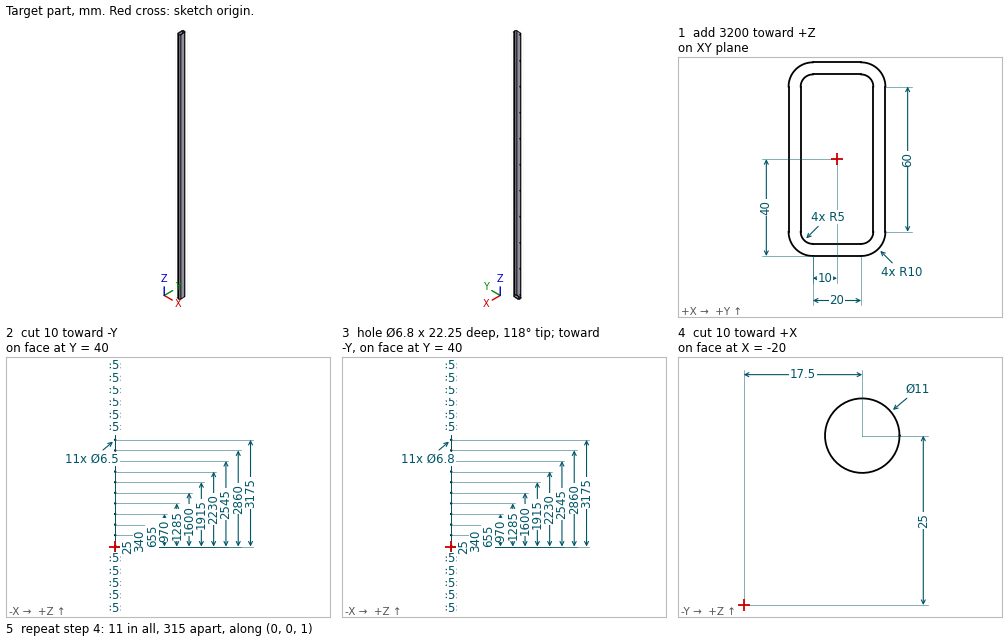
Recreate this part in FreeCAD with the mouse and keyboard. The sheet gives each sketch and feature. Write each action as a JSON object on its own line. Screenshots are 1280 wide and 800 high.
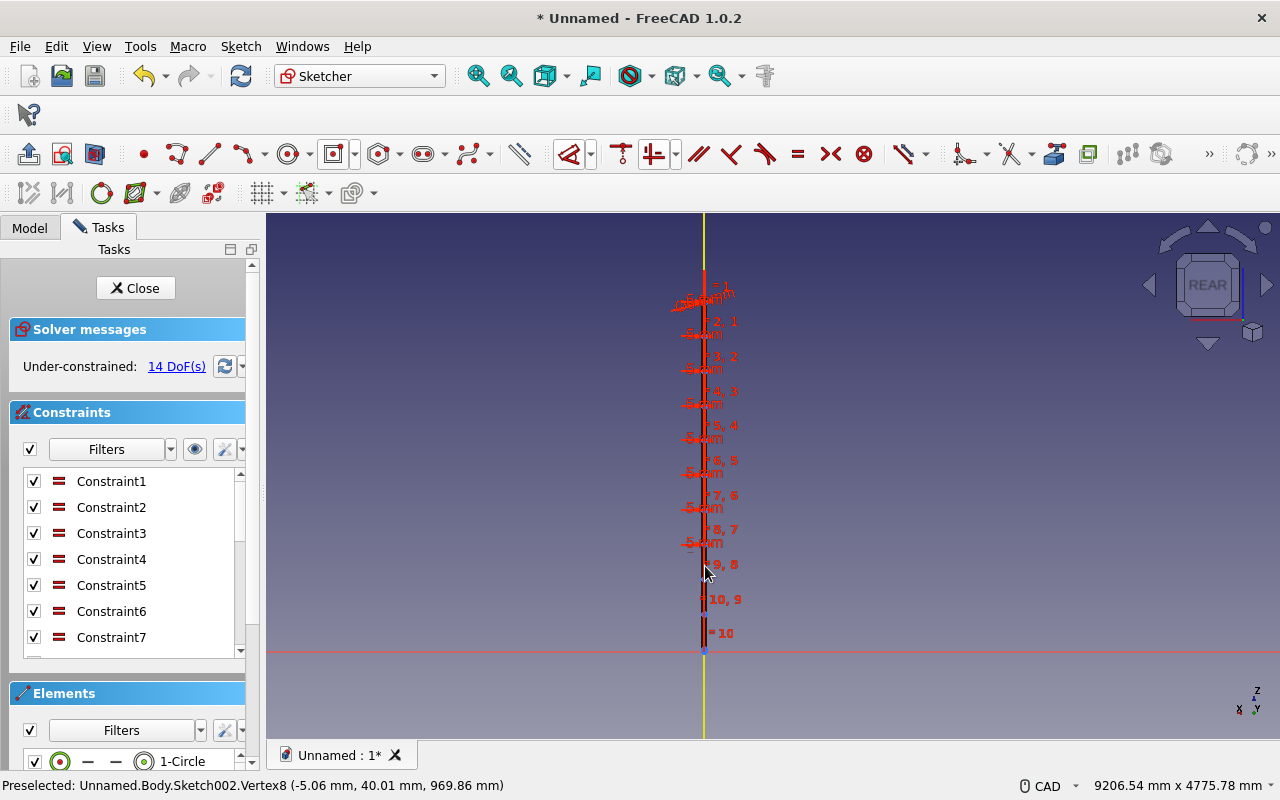
{"action": "scroll", "coordinate": [705, 580], "scroll_direction": "up", "scroll_amount": 22}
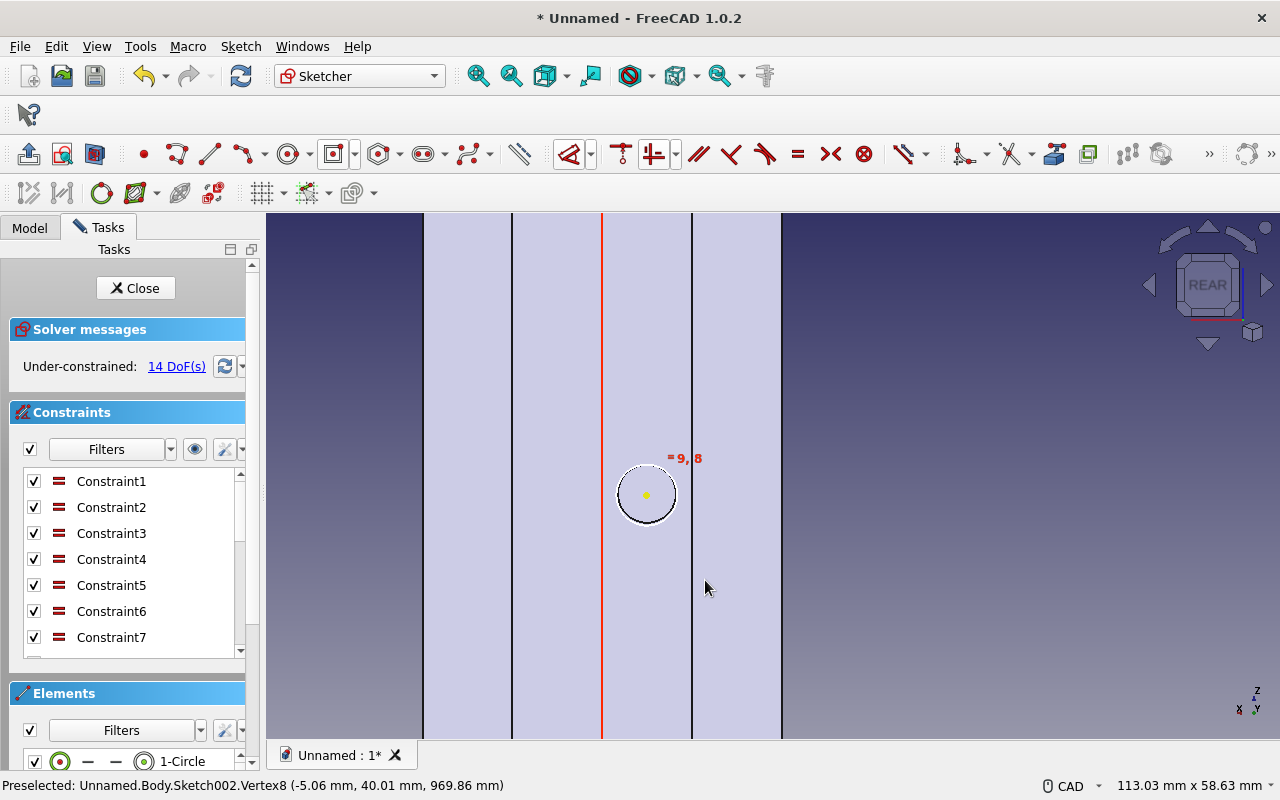
{"action": "left_click", "coordinate": [647, 495]}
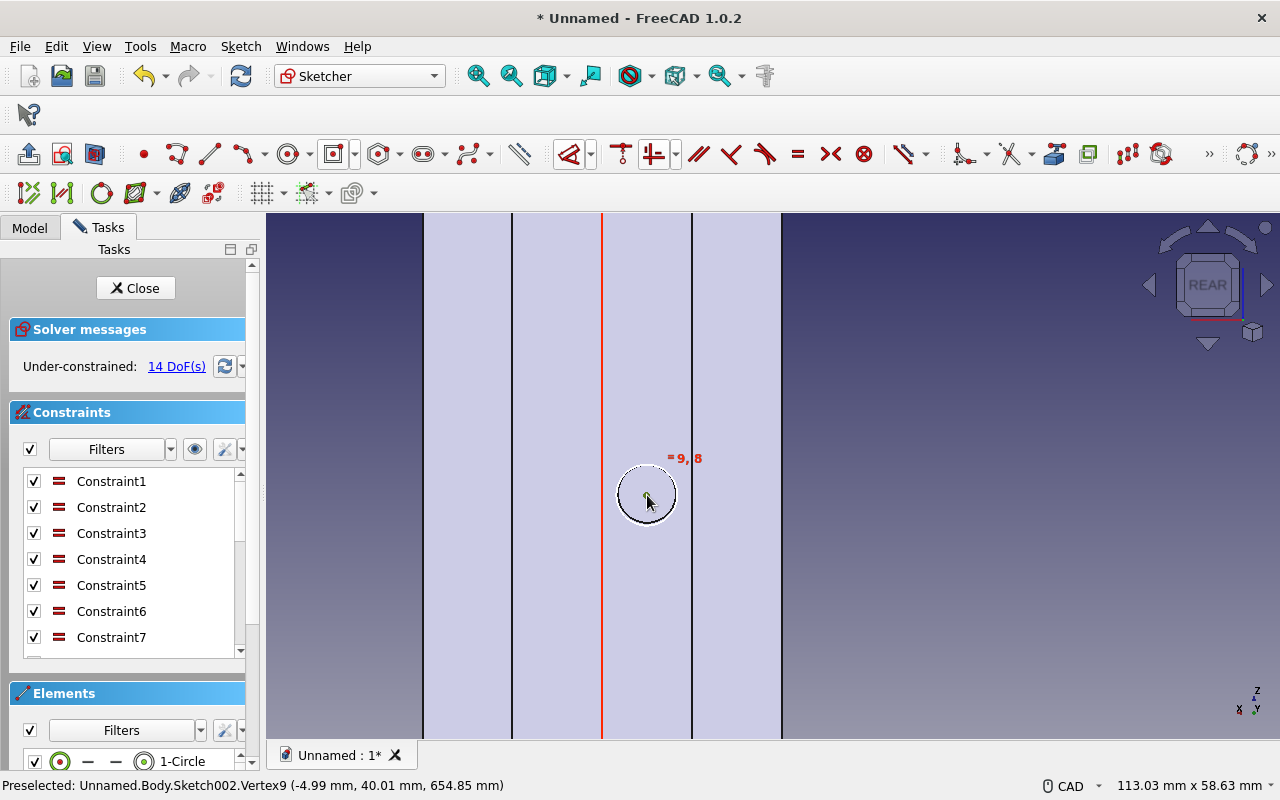
{"action": "key", "text": "l"}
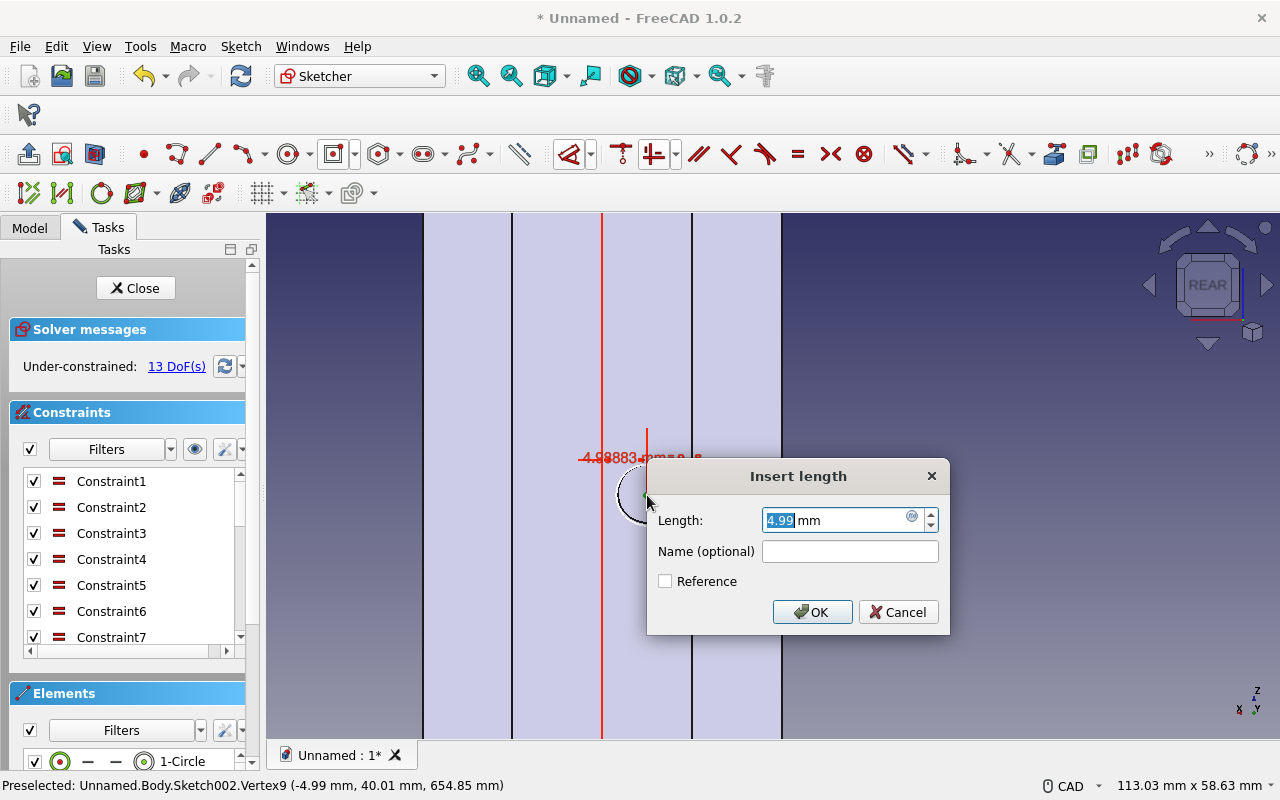
{"action": "type", "text": "5"}
{"action": "key", "text": "Return"}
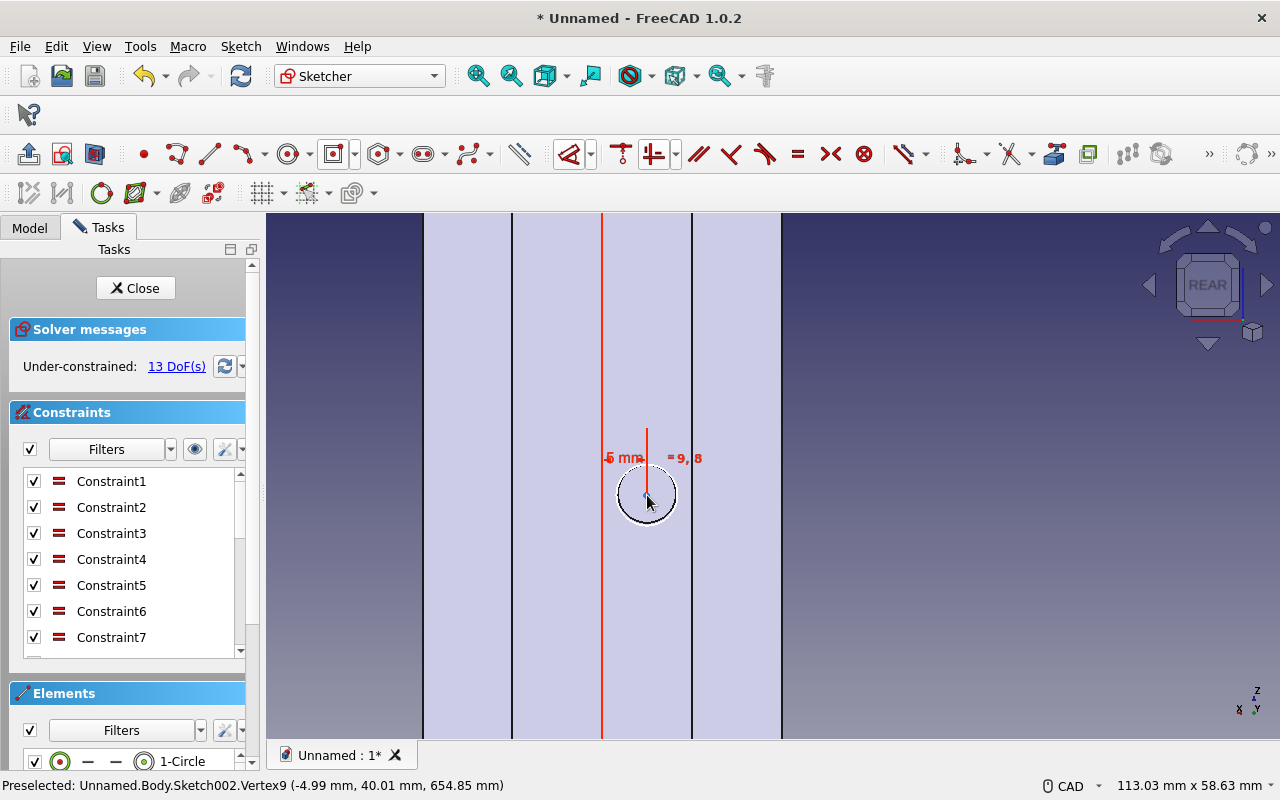
{"action": "scroll", "coordinate": [704, 476], "scroll_direction": "down", "scroll_amount": 15}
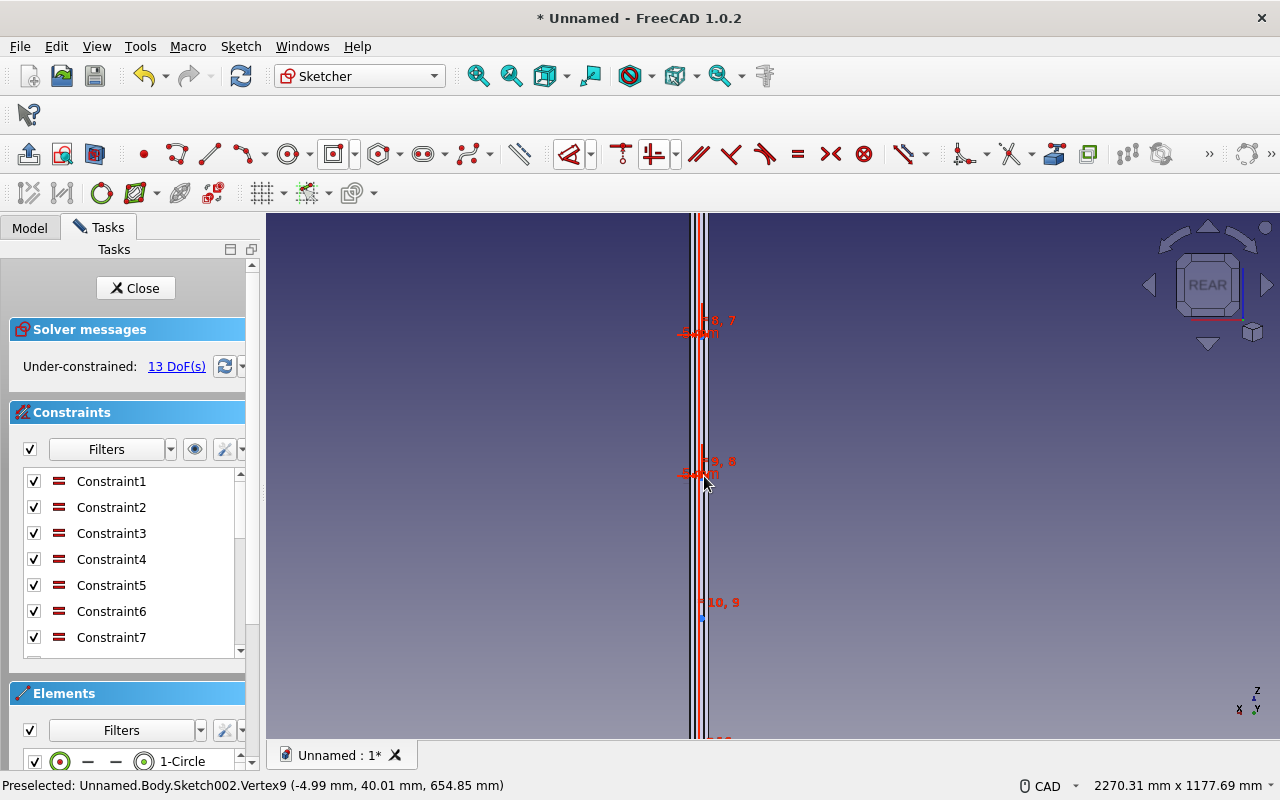
{"action": "scroll", "coordinate": [706, 612], "scroll_direction": "down", "scroll_amount": 7}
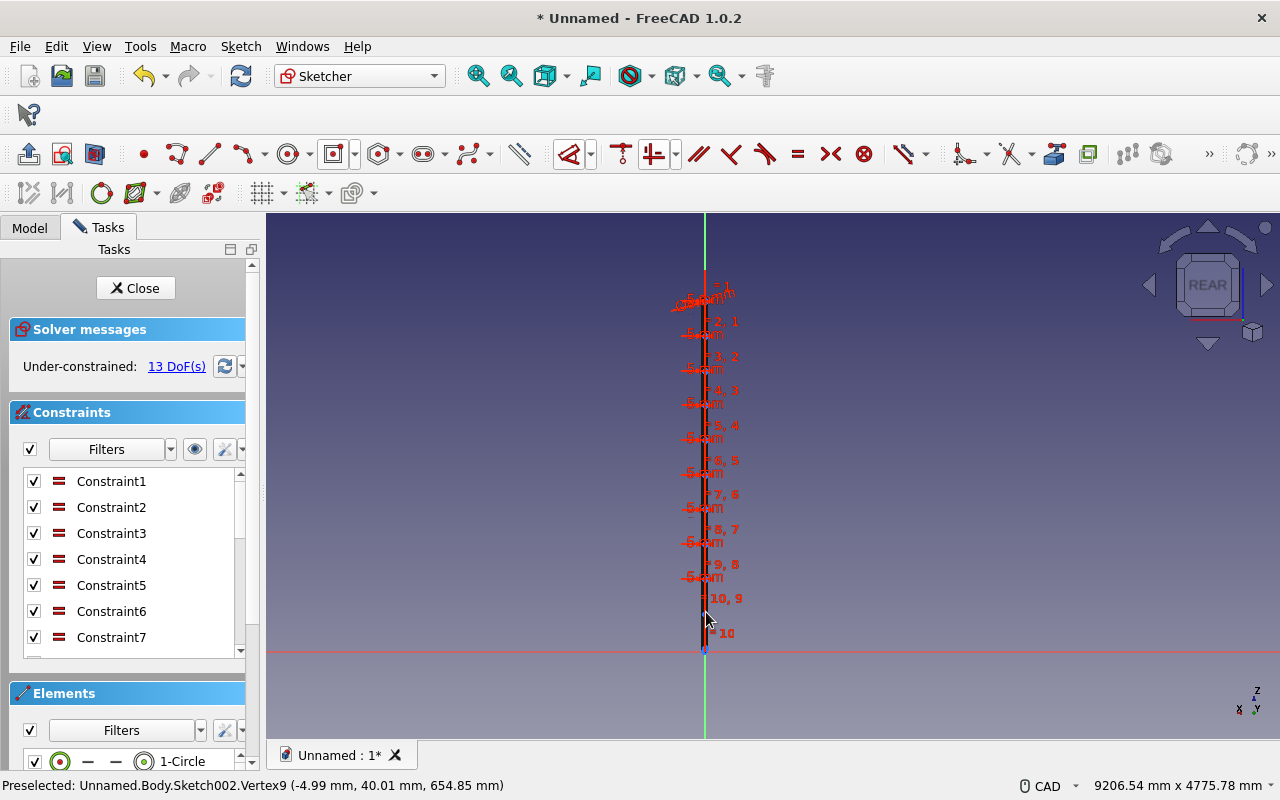
{"action": "scroll", "coordinate": [705, 614], "scroll_direction": "up", "scroll_amount": 22}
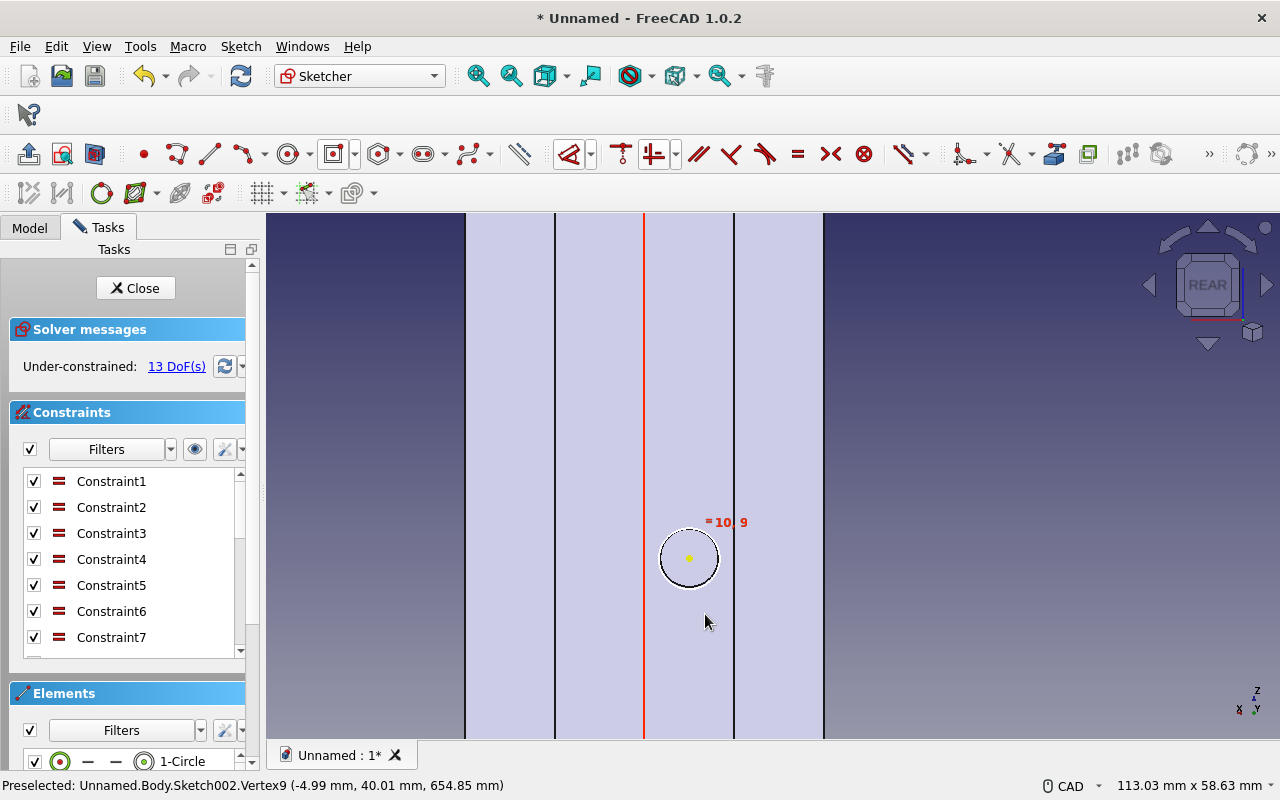
{"action": "left_click", "coordinate": [689, 559]}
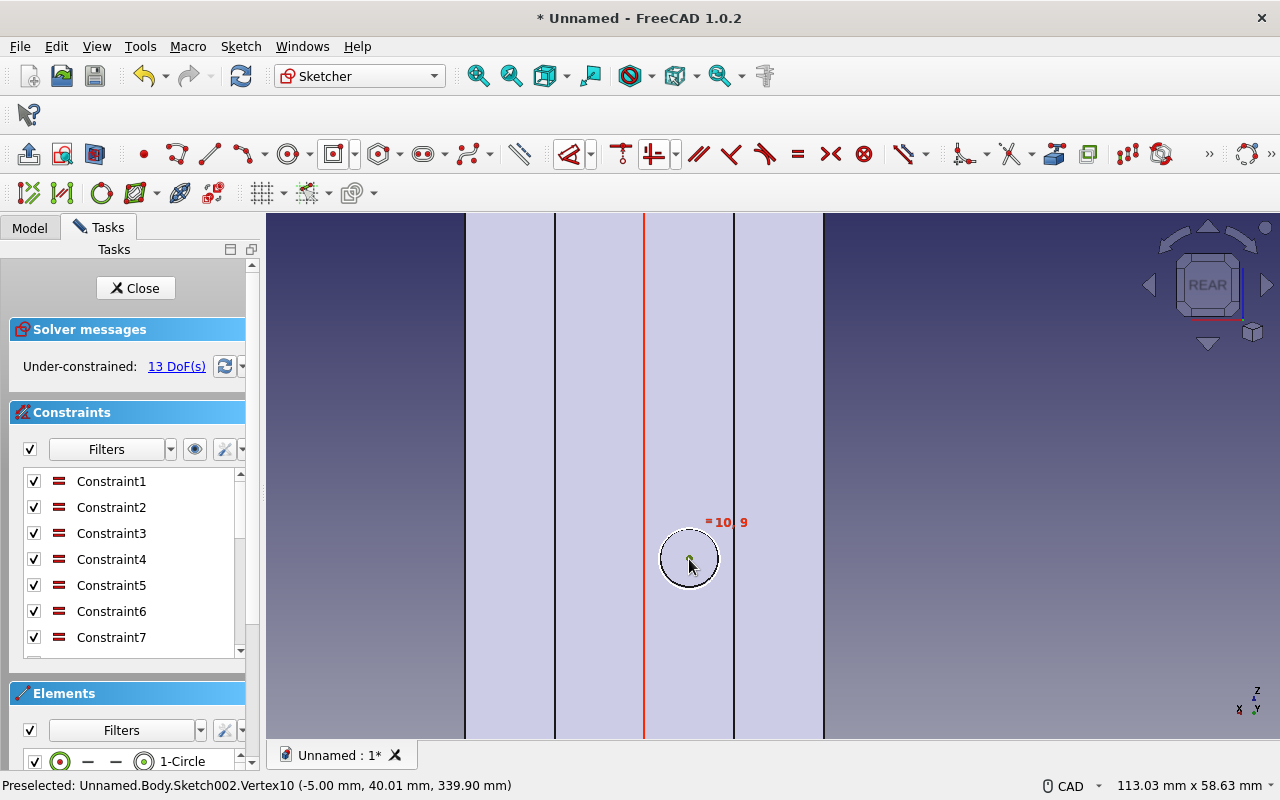
{"action": "key", "text": "l"}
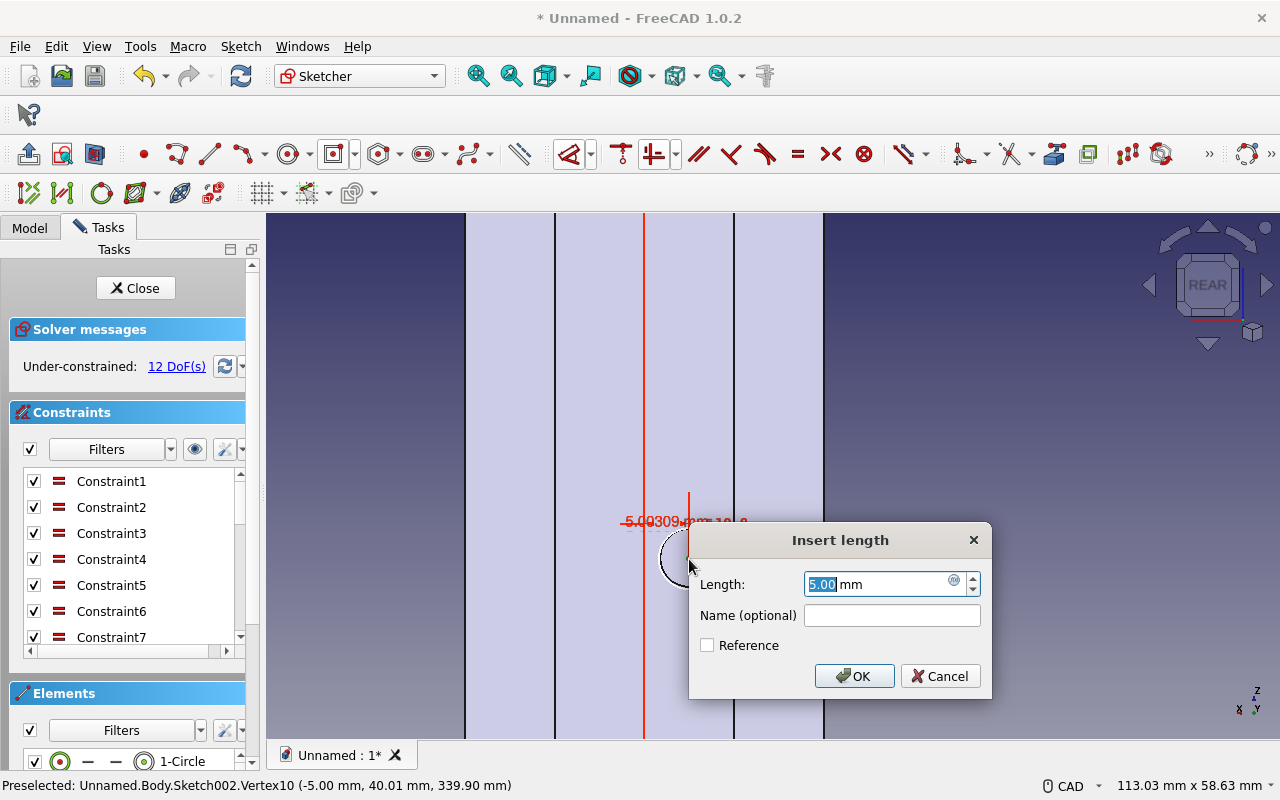
{"action": "type", "text": "5"}
{"action": "key", "text": "Return"}